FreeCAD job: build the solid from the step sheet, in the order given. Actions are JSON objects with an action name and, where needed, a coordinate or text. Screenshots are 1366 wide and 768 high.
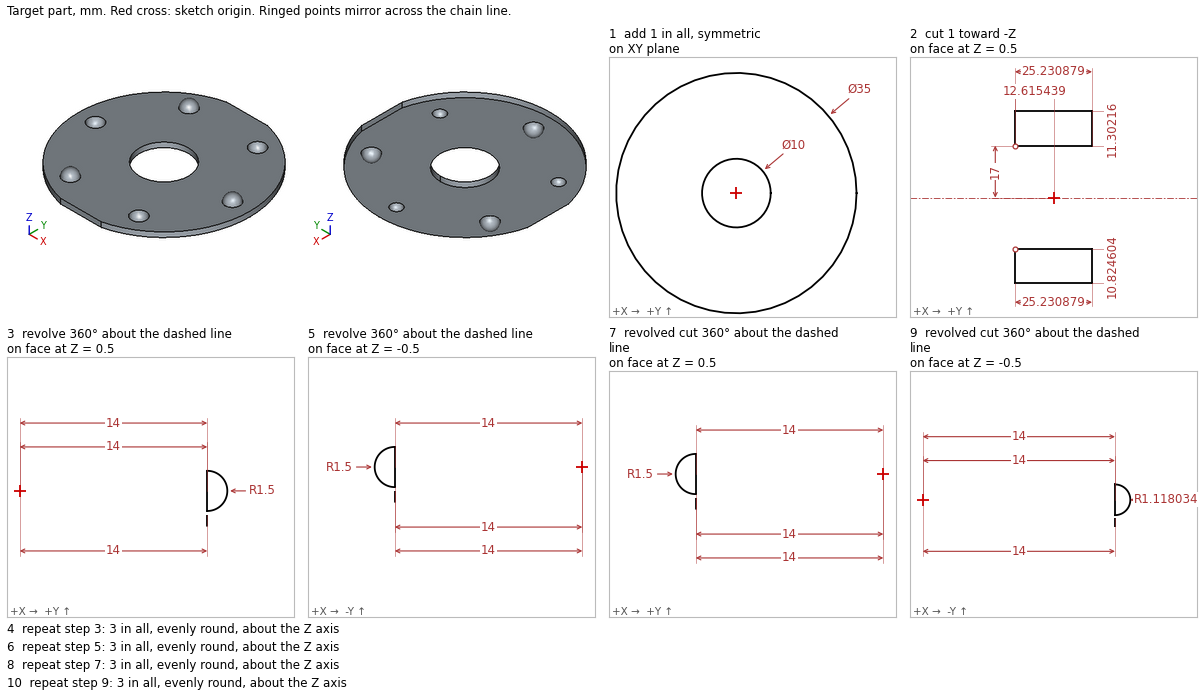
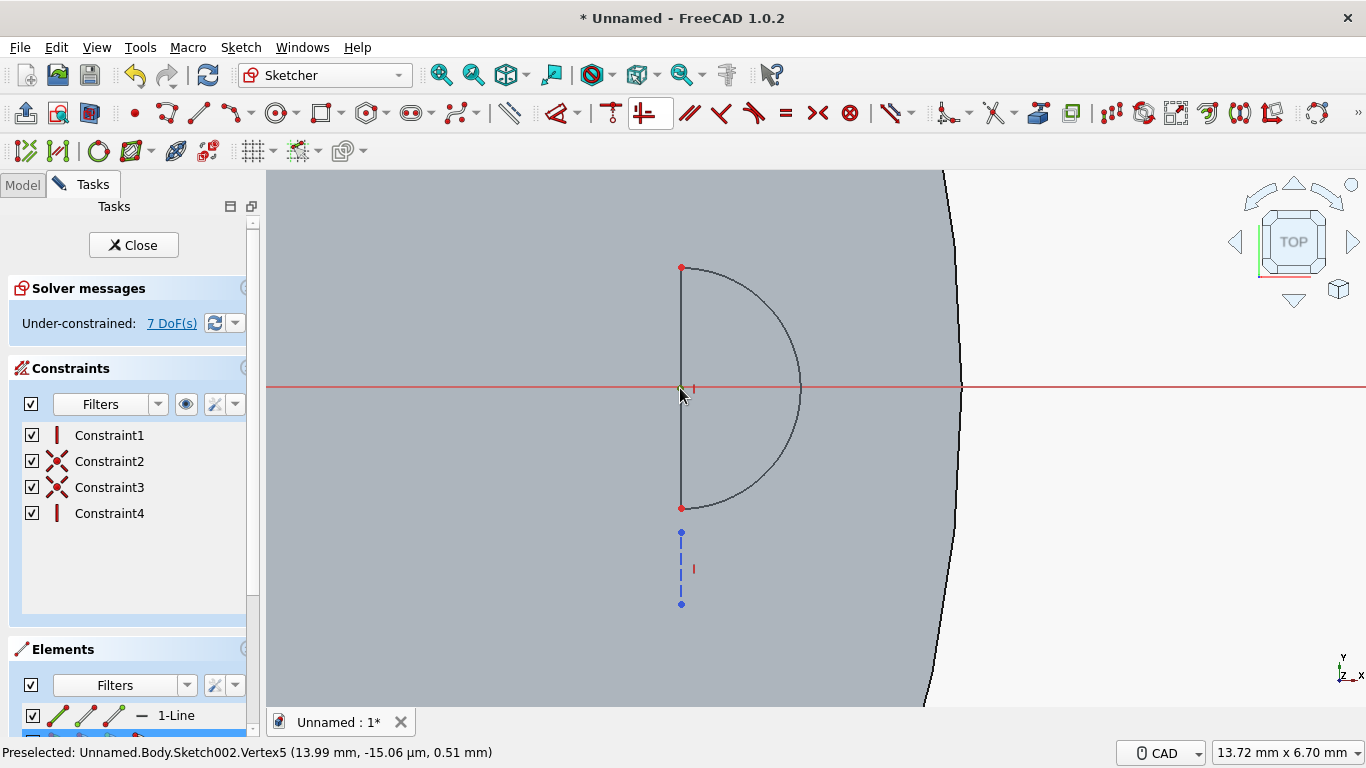
{"action": "left_click", "coordinate": [359, 387]}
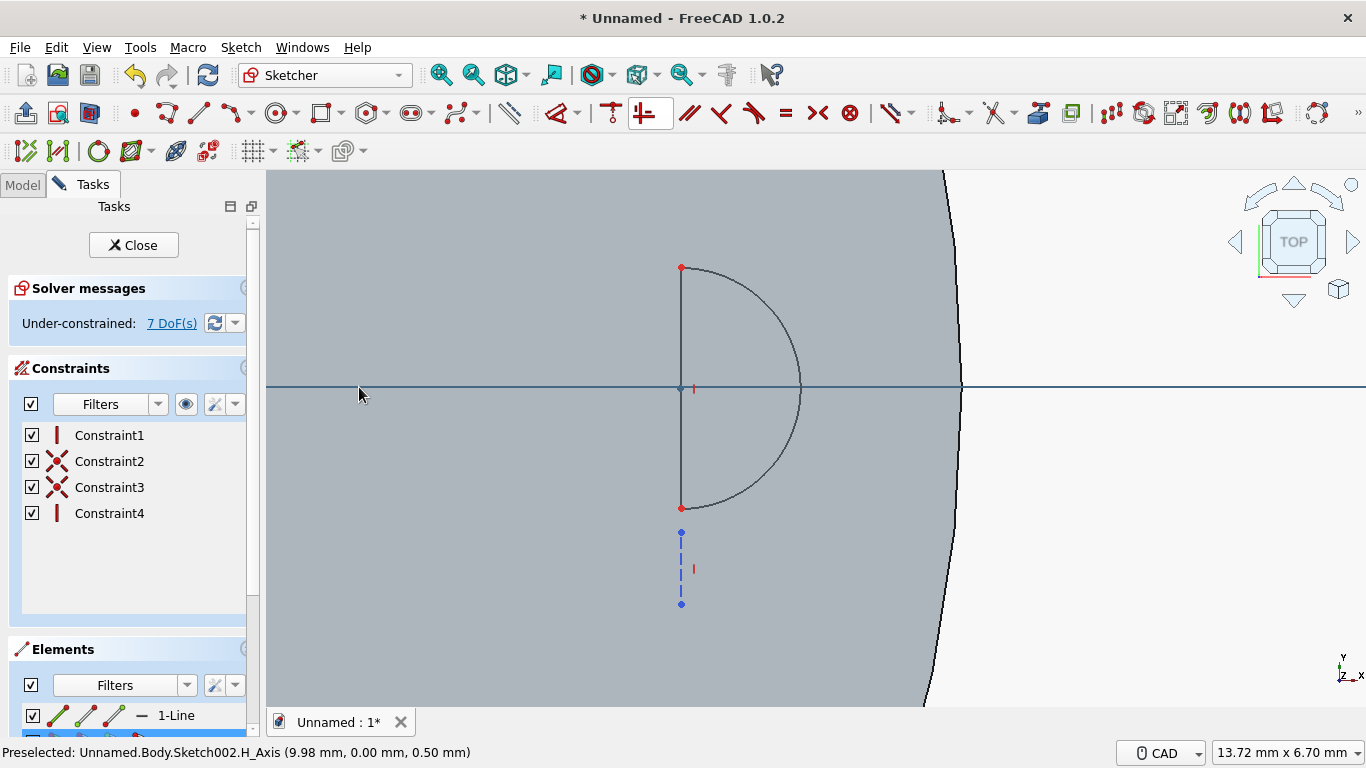
{"action": "key", "text": "c"}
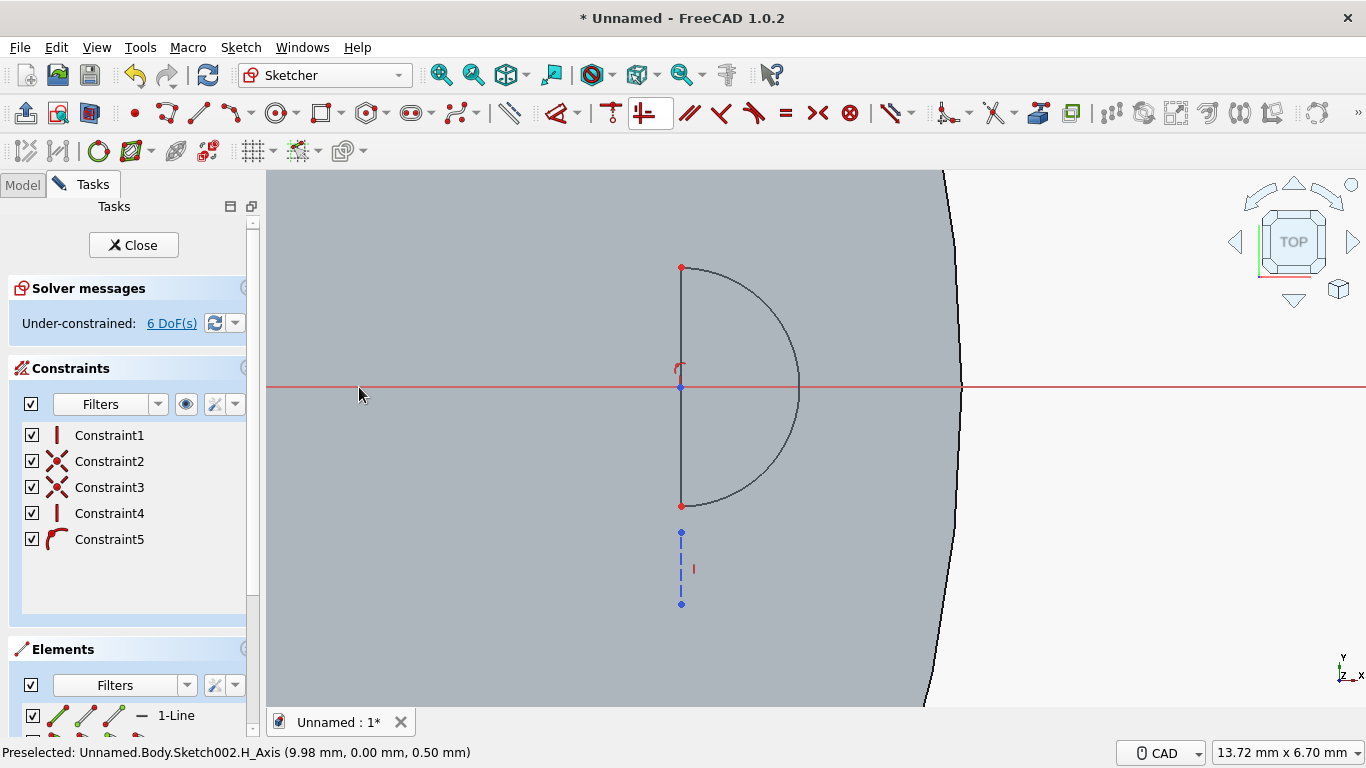
{"action": "key", "text": "d"}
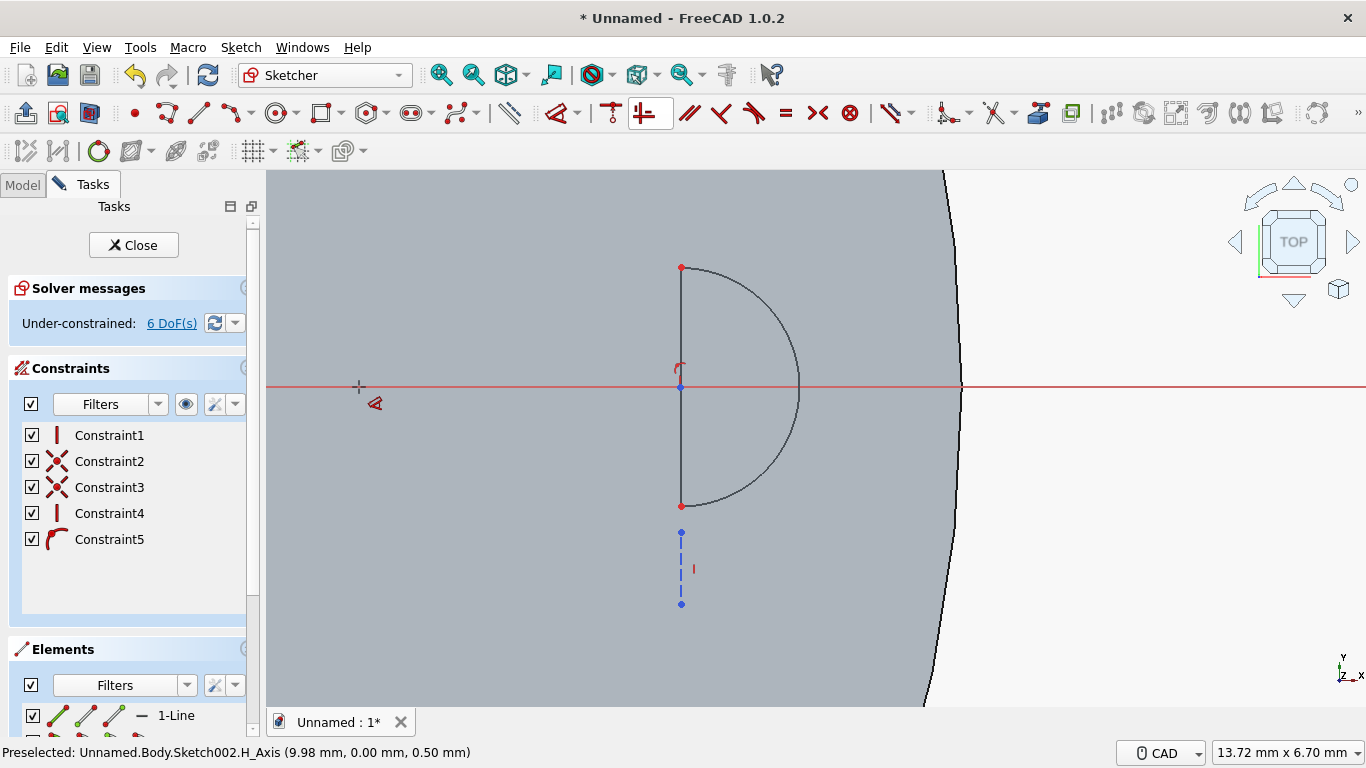
{"action": "left_click", "coordinate": [777, 457]}
{"action": "left_click", "coordinate": [803, 476]}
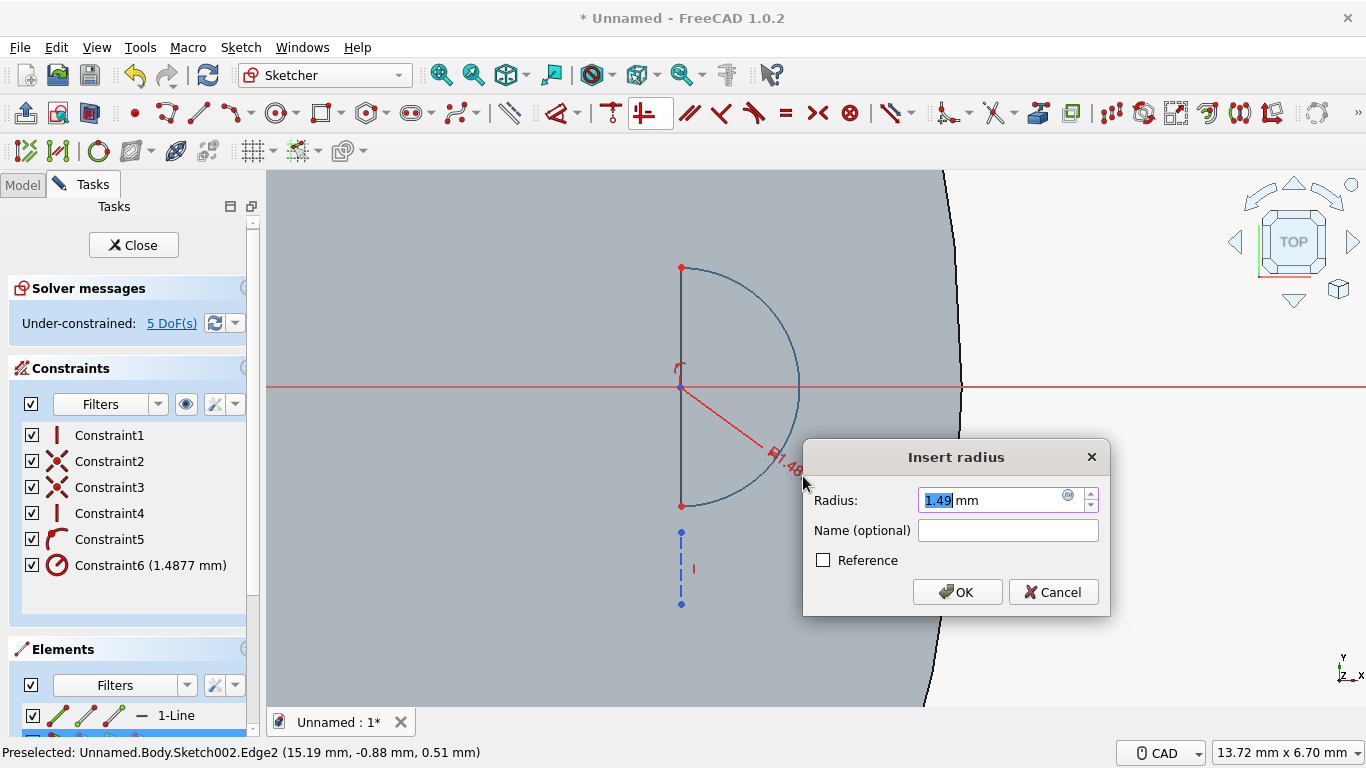
{"action": "type", "text": "1.5"}
{"action": "key", "text": "Return"}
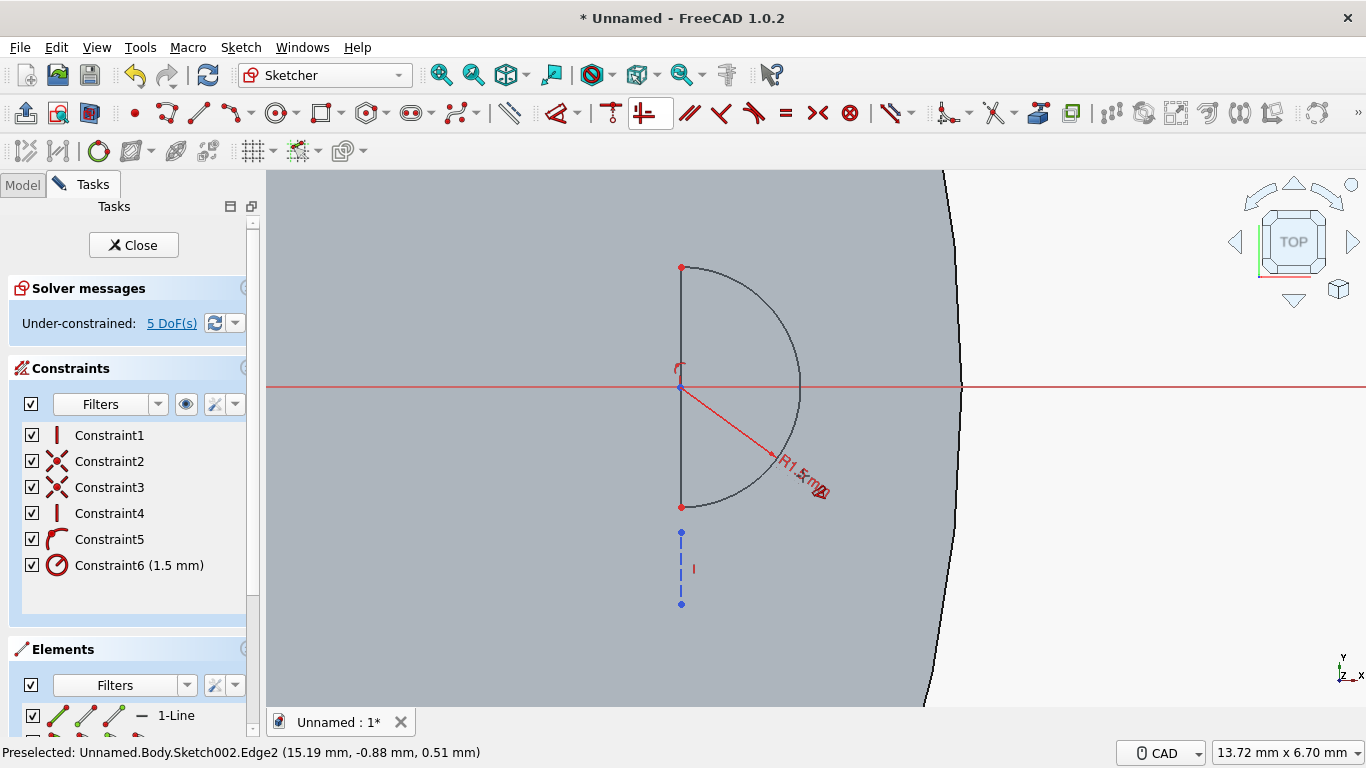
{"action": "left_click", "coordinate": [681, 267]}
{"action": "left_click", "coordinate": [488, 233]}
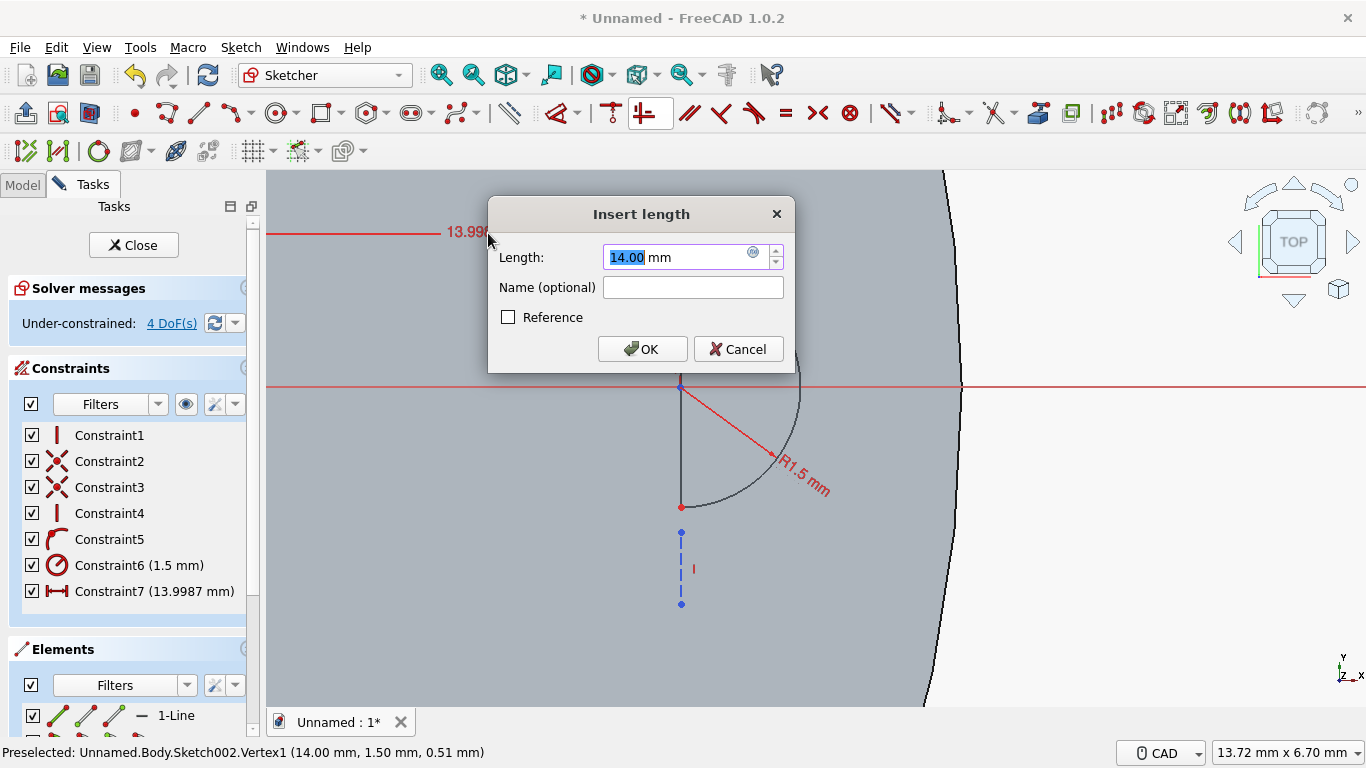
{"action": "type", "text": "14"}
{"action": "key", "text": "Return"}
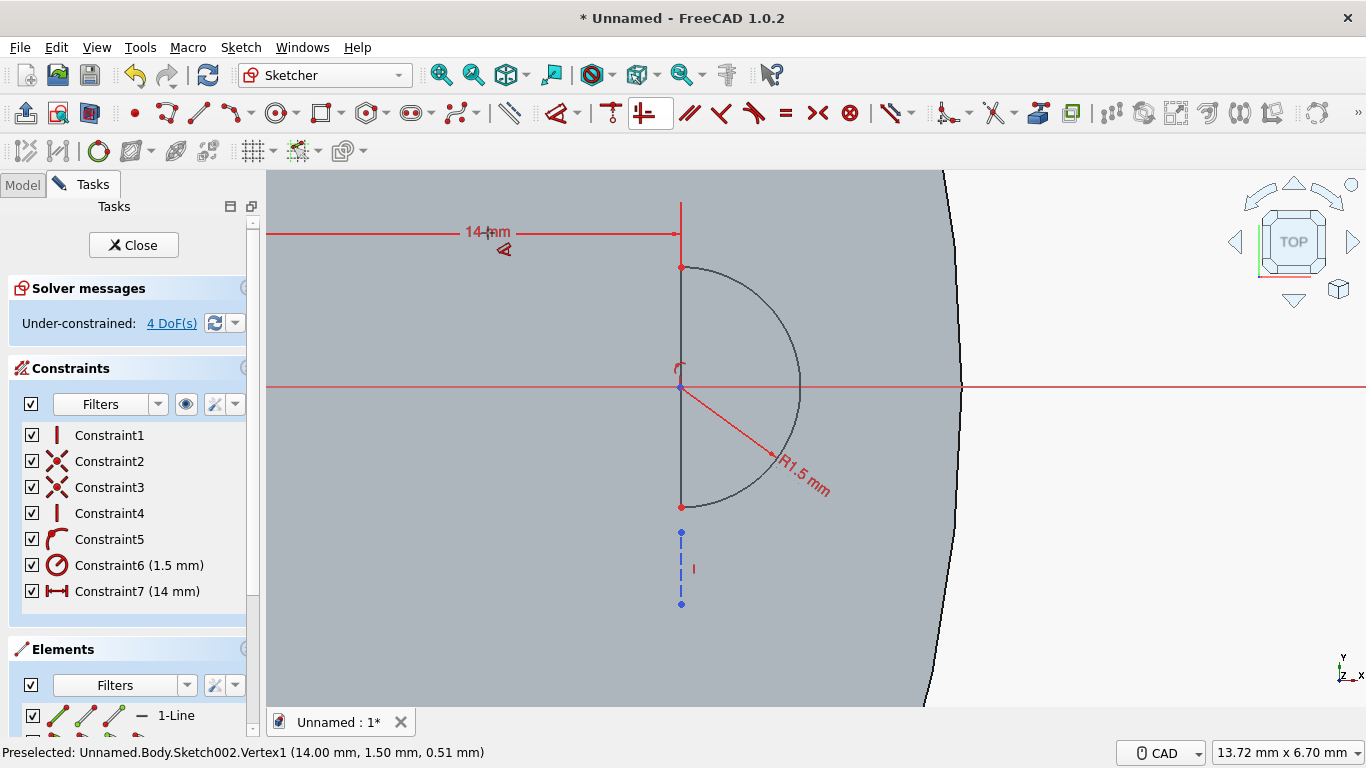
{"action": "left_click", "coordinate": [681, 533]}
{"action": "left_click", "coordinate": [487, 567]}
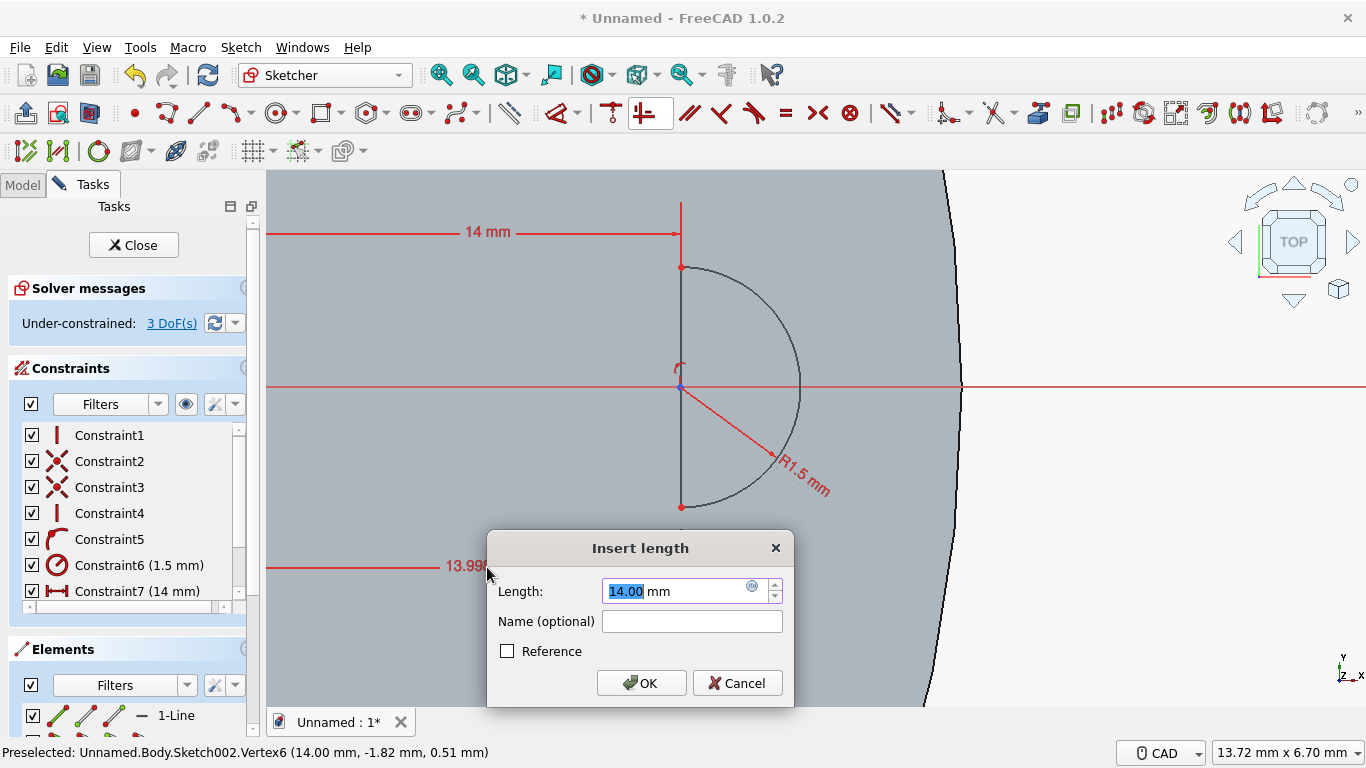
{"action": "type", "text": "14"}
{"action": "key", "text": "Return"}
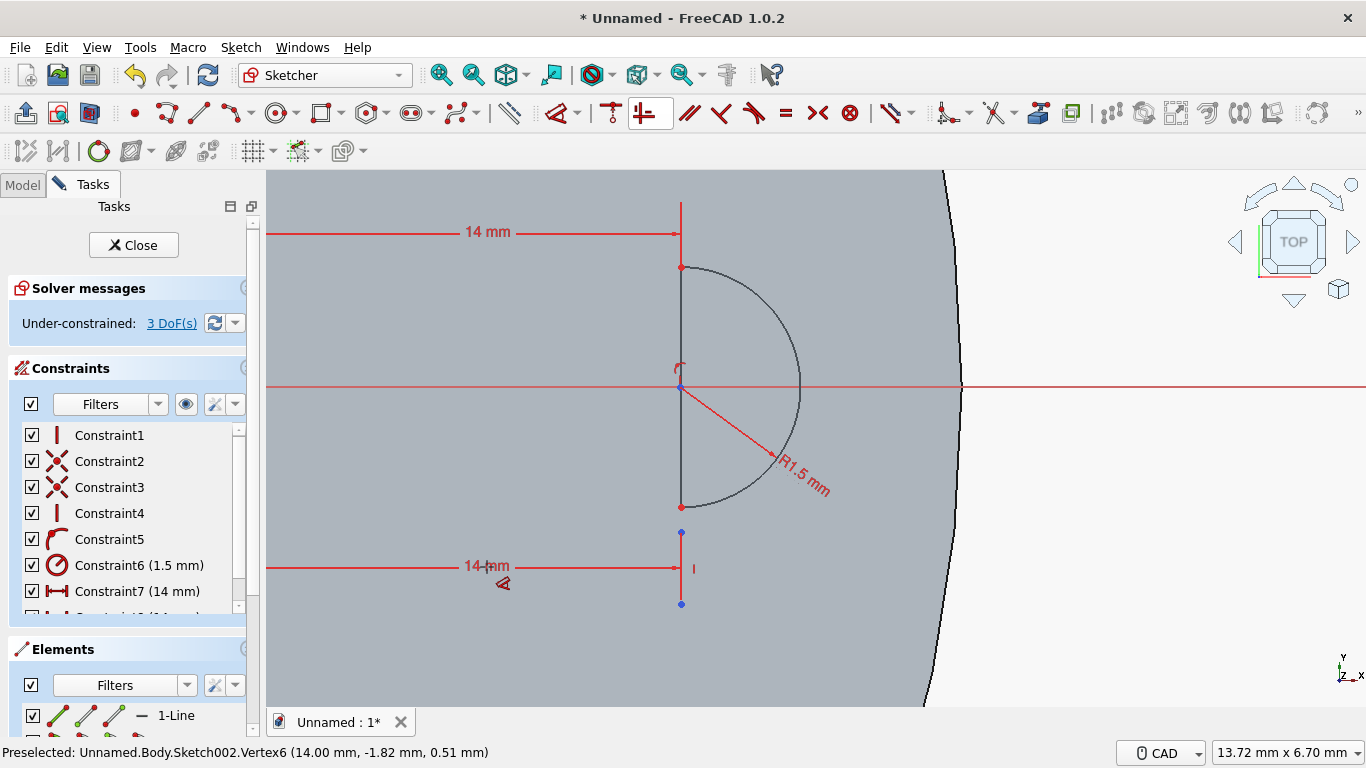
{"action": "left_click", "coordinate": [680, 387]}
{"action": "left_click", "coordinate": [487, 353]}